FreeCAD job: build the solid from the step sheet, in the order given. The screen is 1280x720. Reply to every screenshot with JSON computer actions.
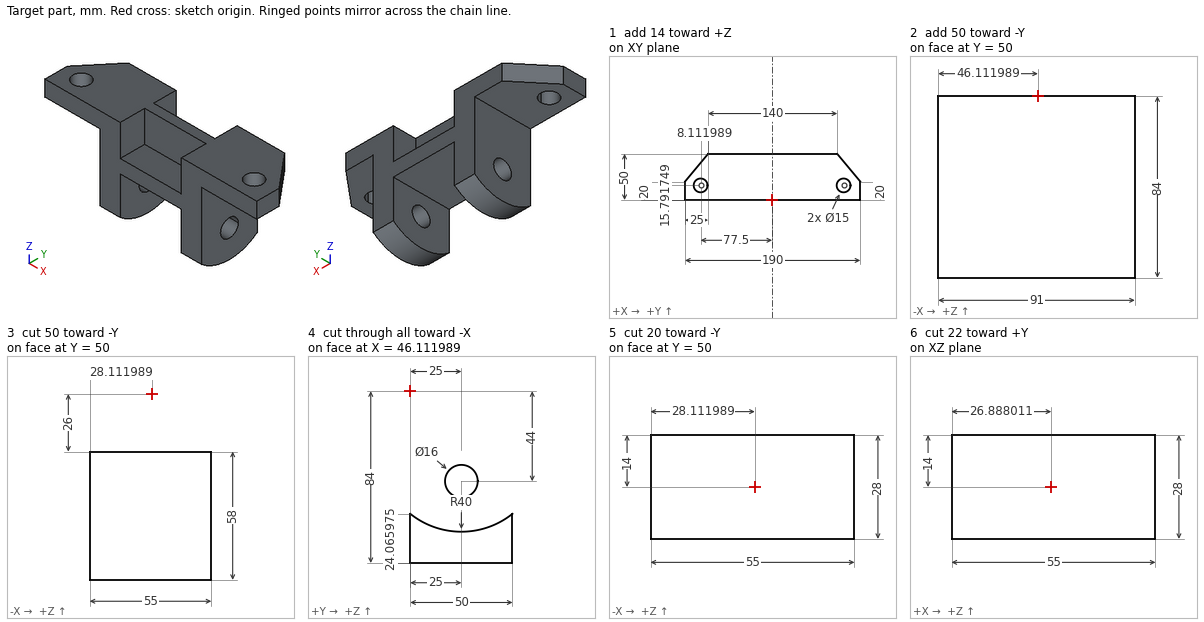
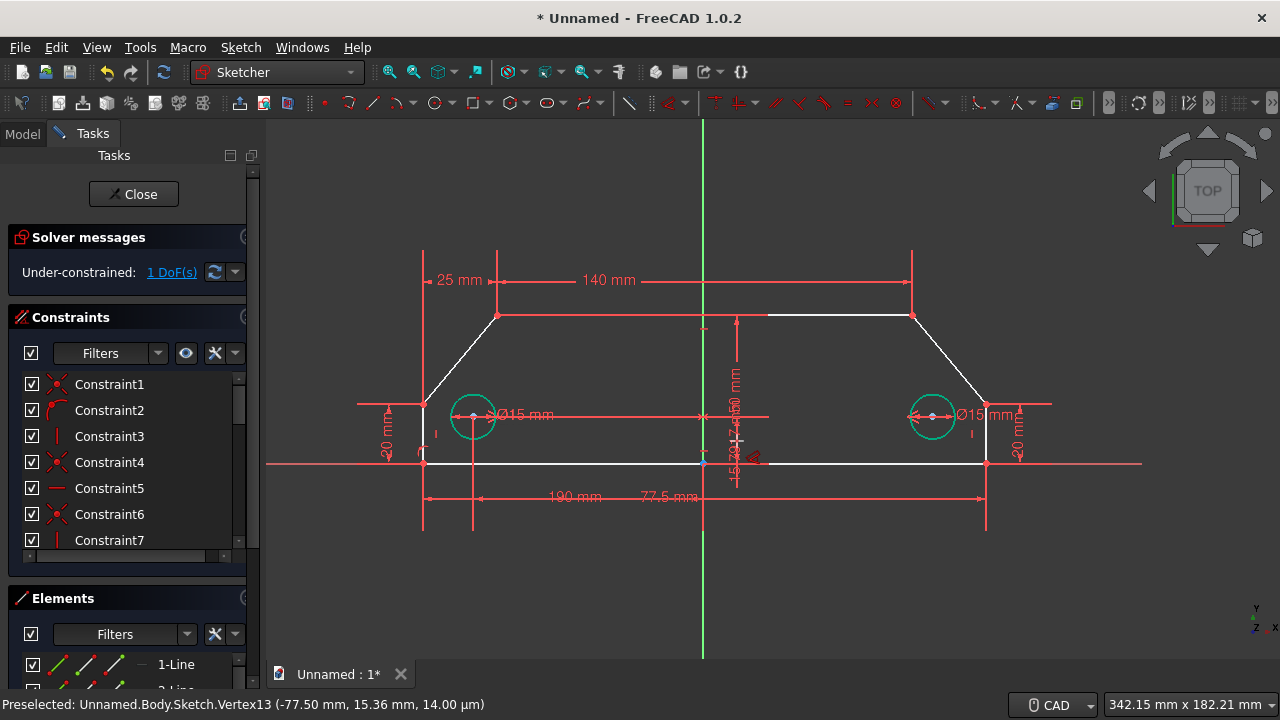
{"action": "scroll", "coordinate": [497, 315], "scroll_direction": "up", "scroll_amount": 3}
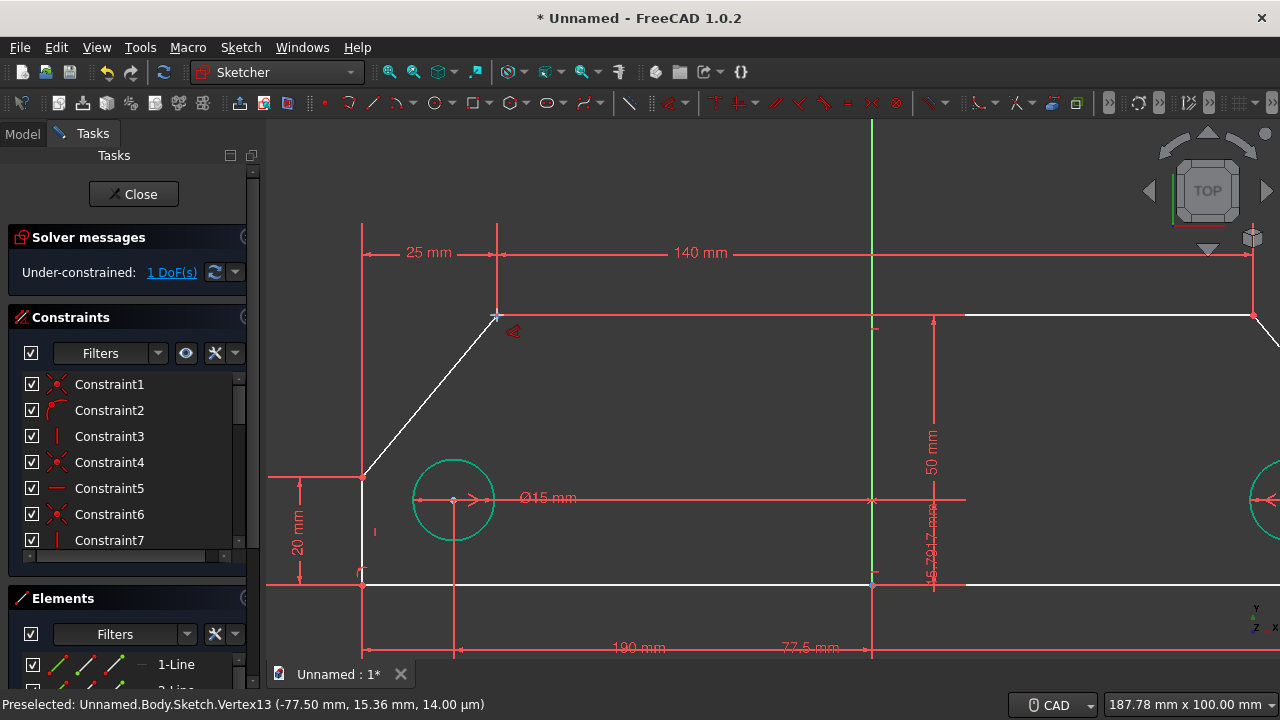
{"action": "left_click", "coordinate": [497, 315]}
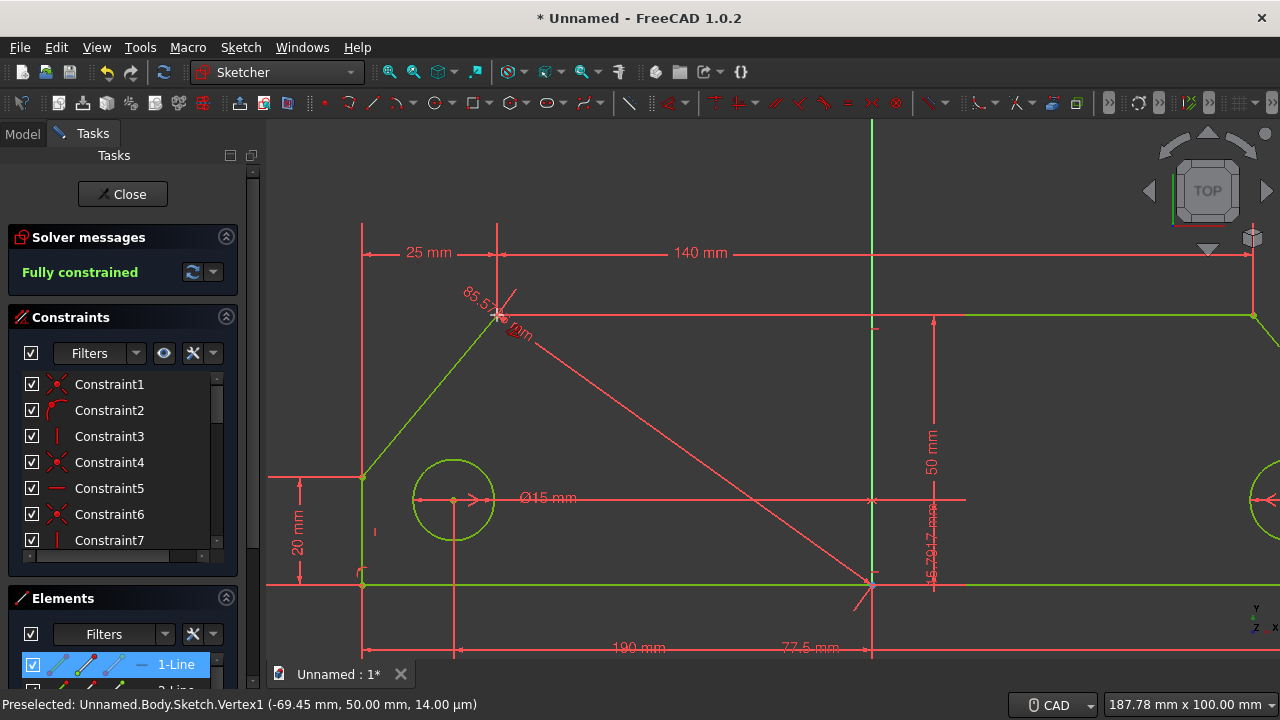
{"action": "left_click", "coordinate": [454, 500]}
{"action": "left_click", "coordinate": [475, 281]}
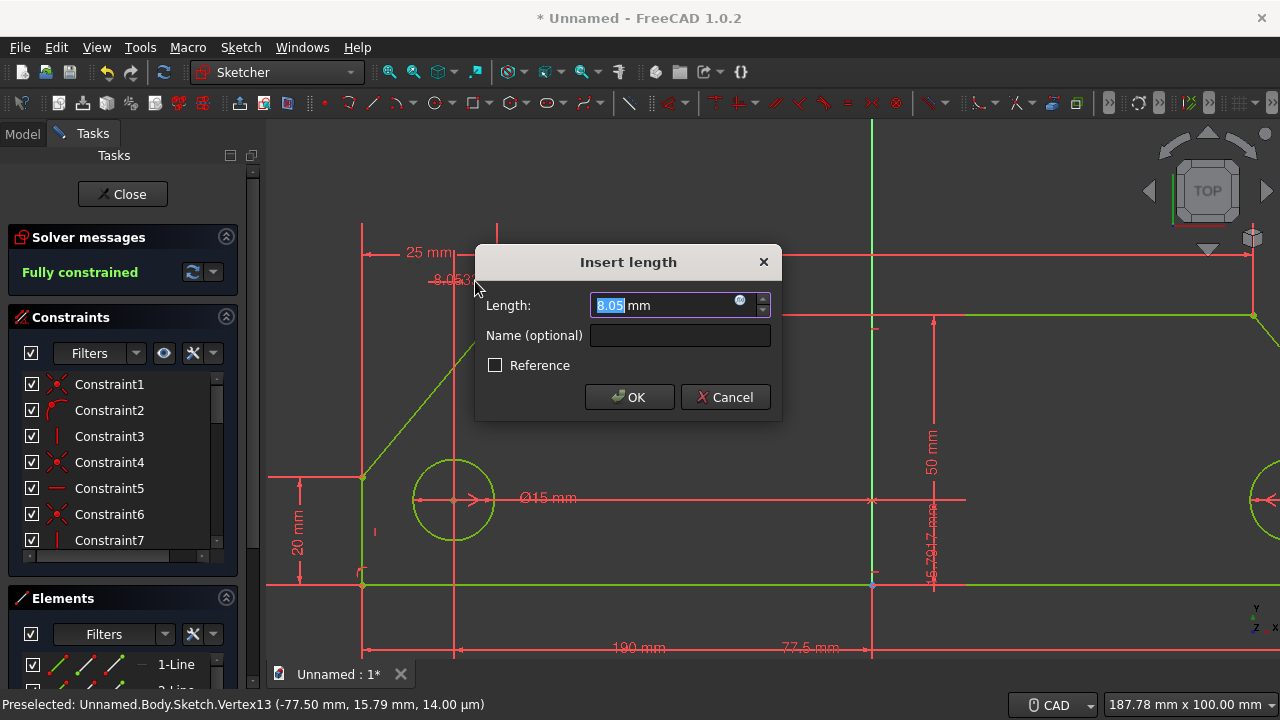
{"action": "type", "text": "8.111989"}
{"action": "key", "text": "Return"}
{"action": "key", "text": "Escape"}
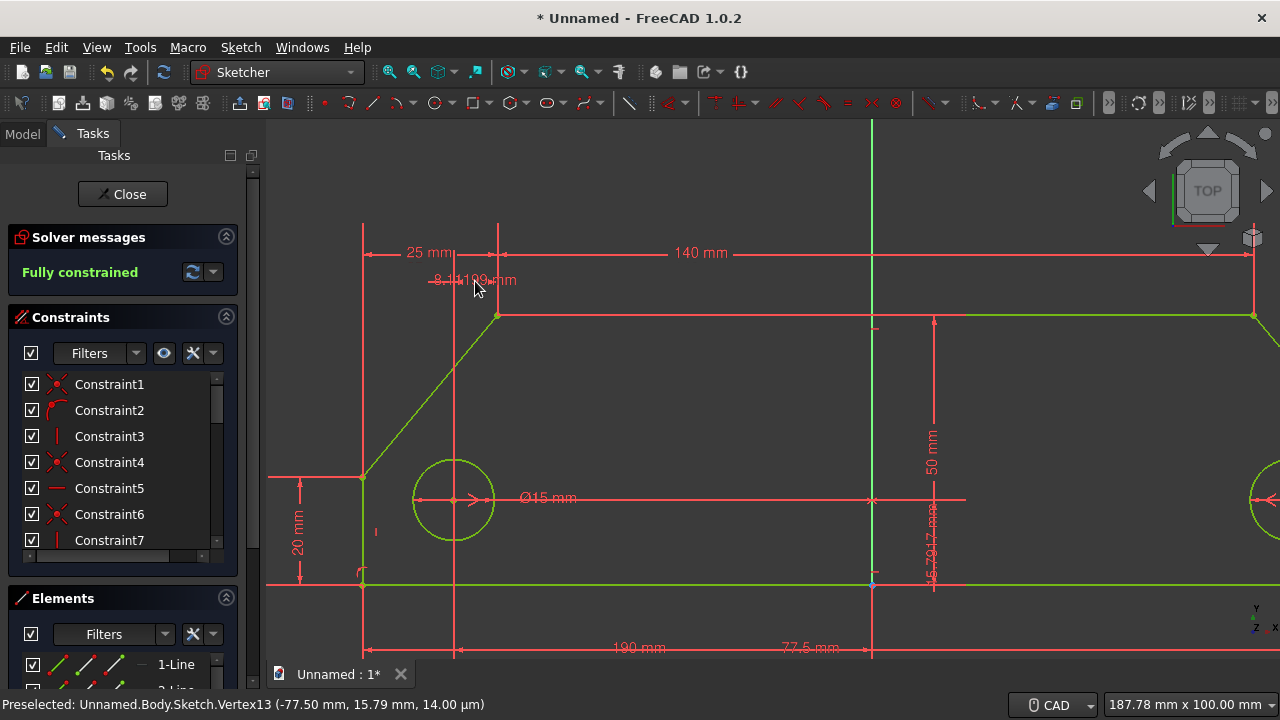
{"action": "left_click", "coordinate": [123, 194]}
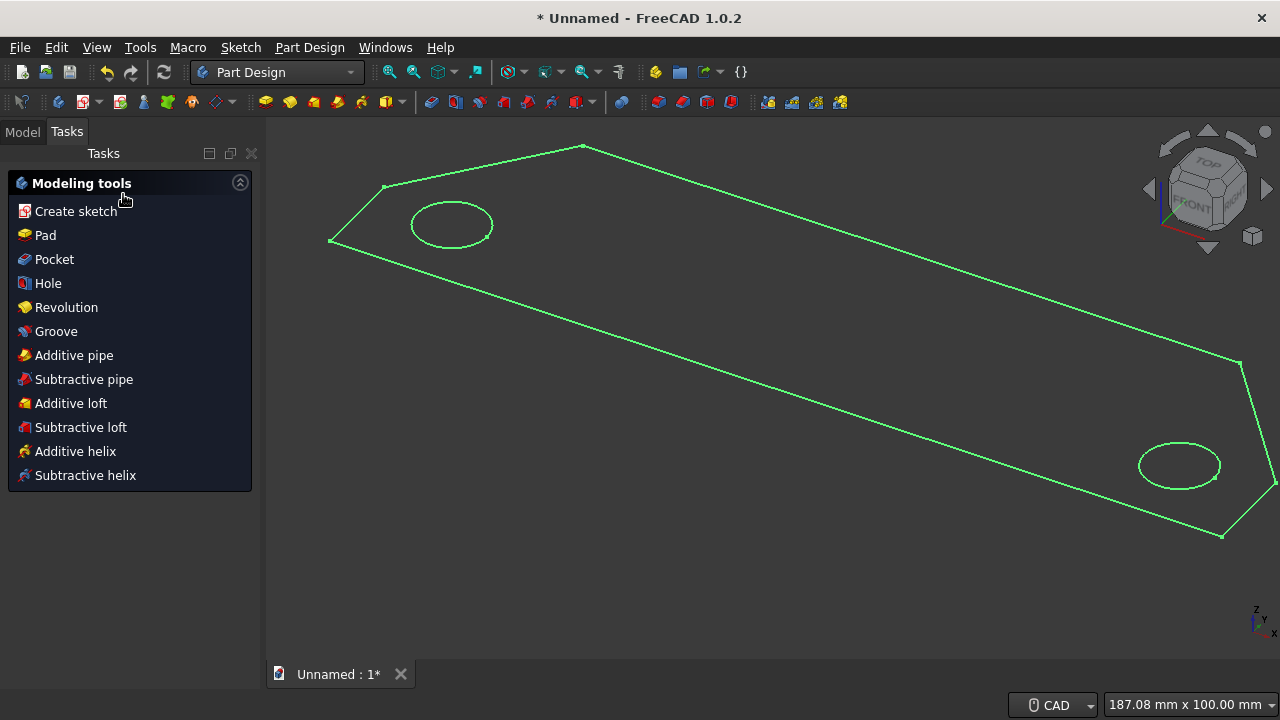
{"action": "left_click", "coordinate": [266, 102]}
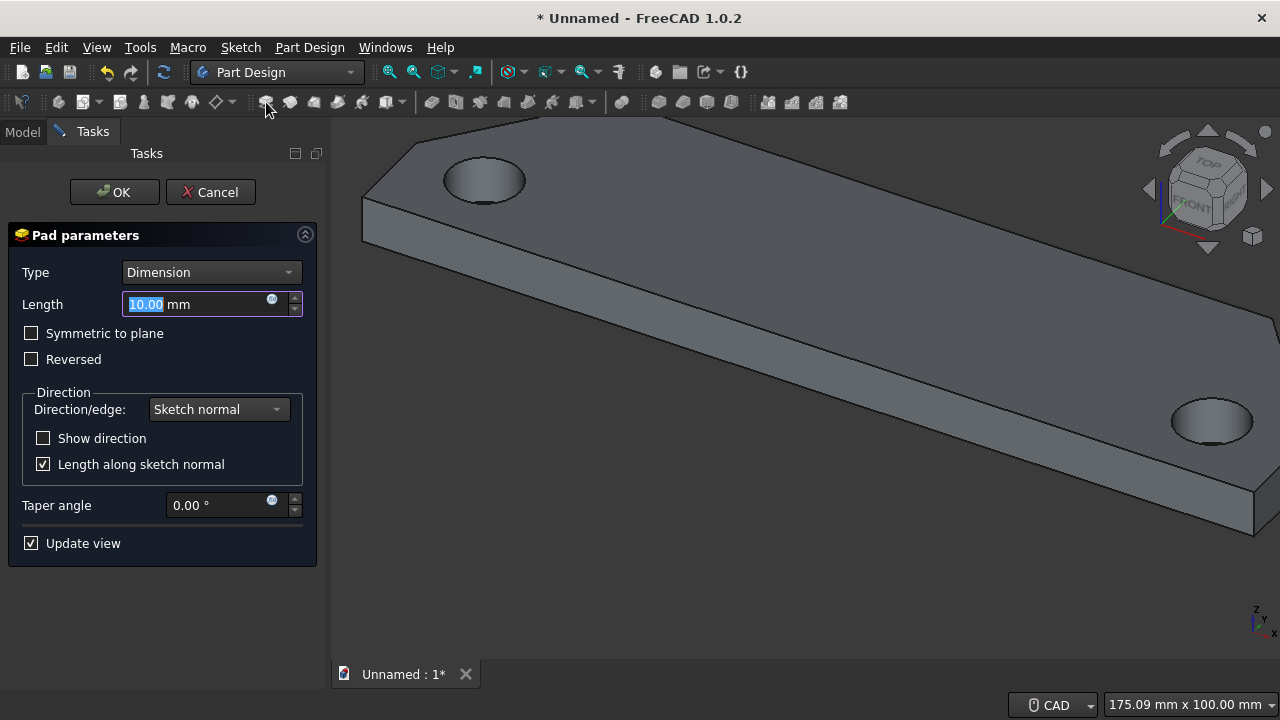
{"action": "type", "text": "14"}
{"action": "key", "text": "Tab"}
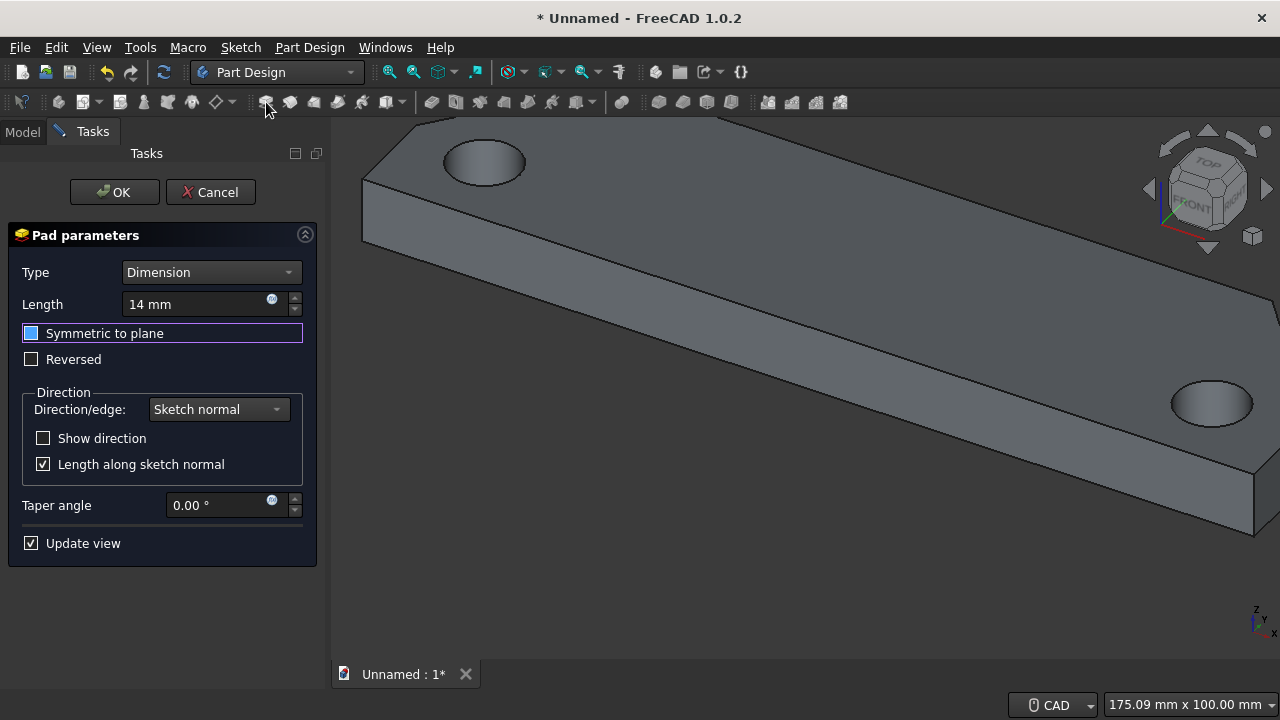
{"action": "left_click", "coordinate": [115, 192]}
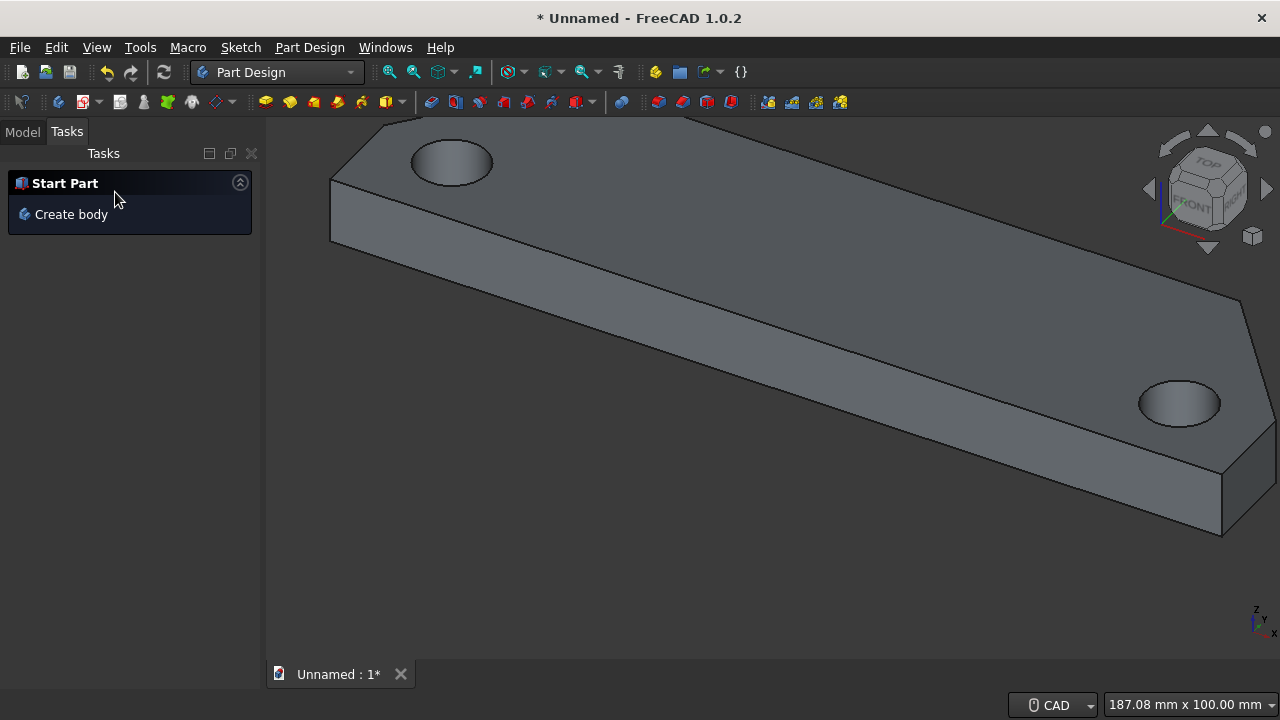
{"action": "left_click", "coordinate": [390, 72]}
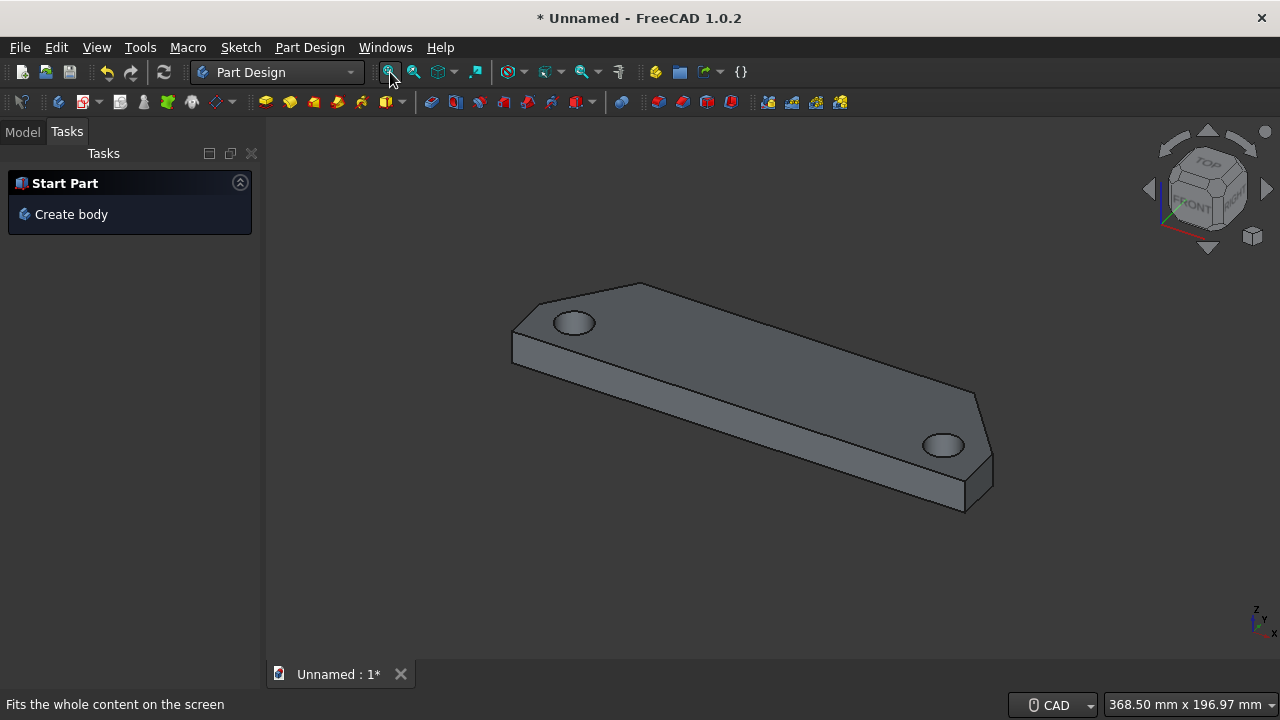
{"action": "key", "text": "4"}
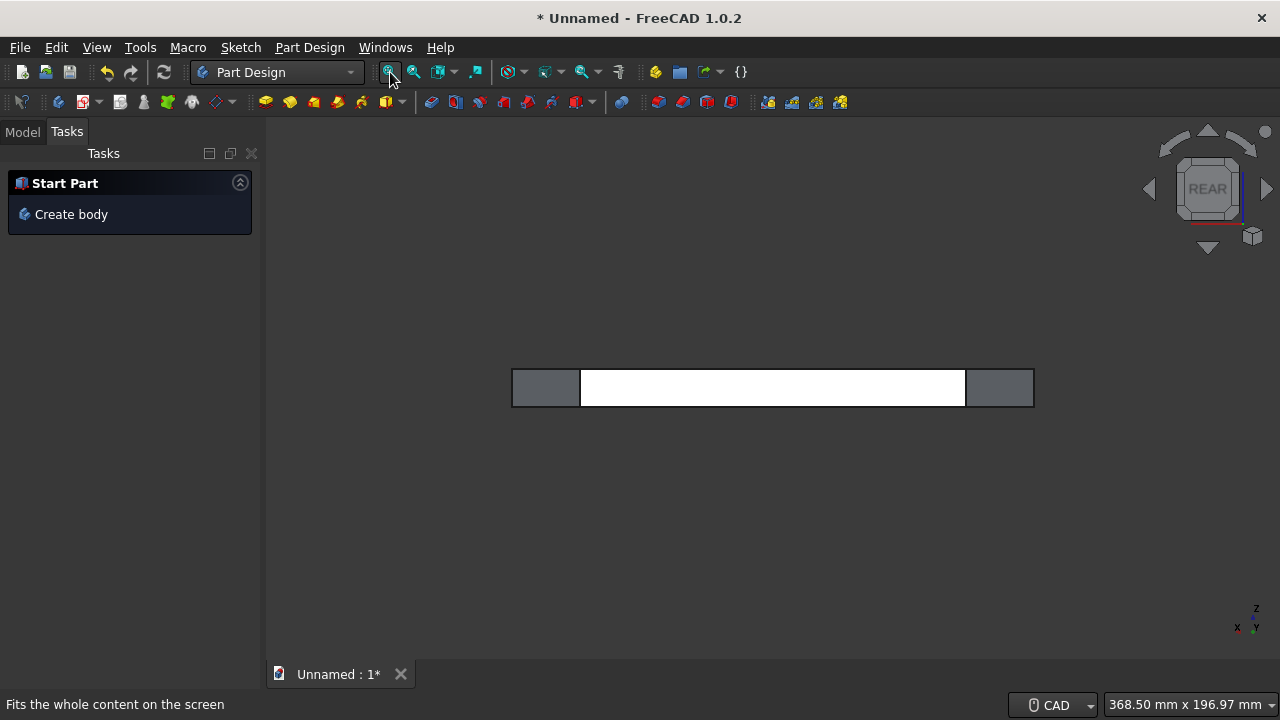
{"action": "left_click", "coordinate": [608, 387]}